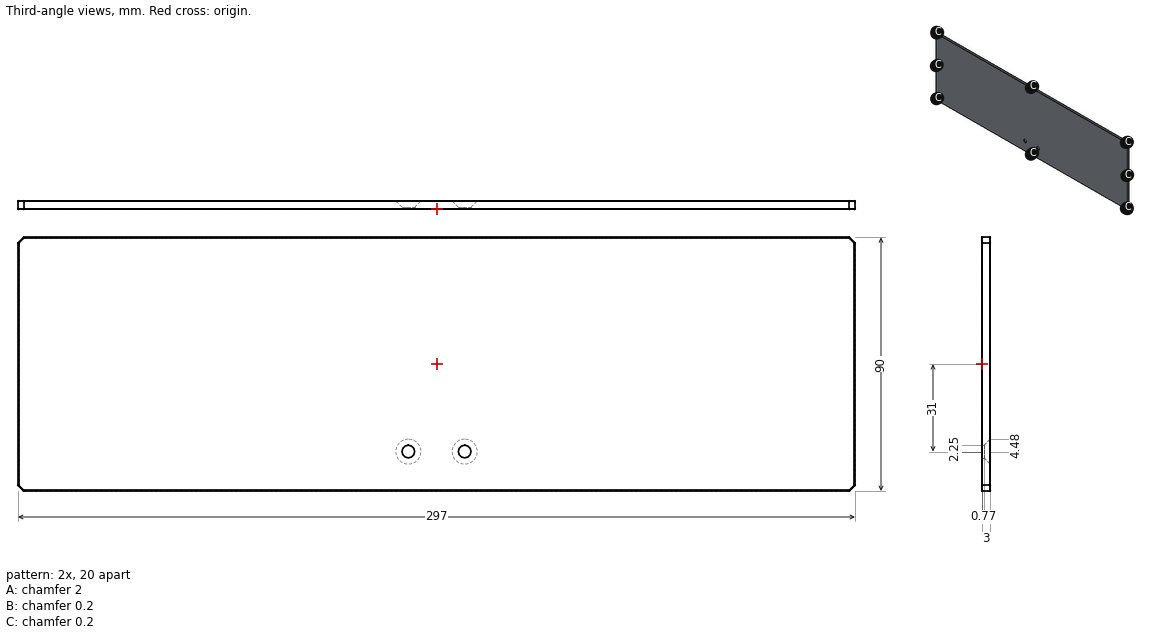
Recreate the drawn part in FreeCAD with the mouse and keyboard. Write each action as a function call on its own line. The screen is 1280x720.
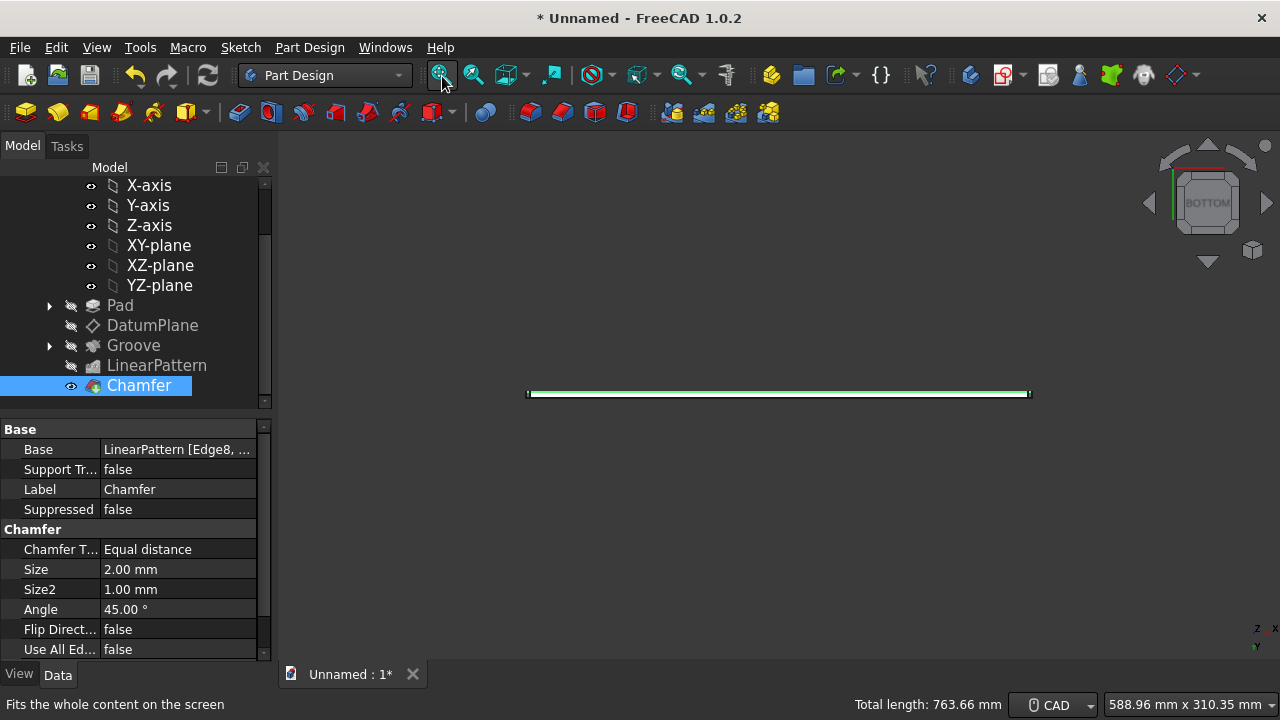
key(4)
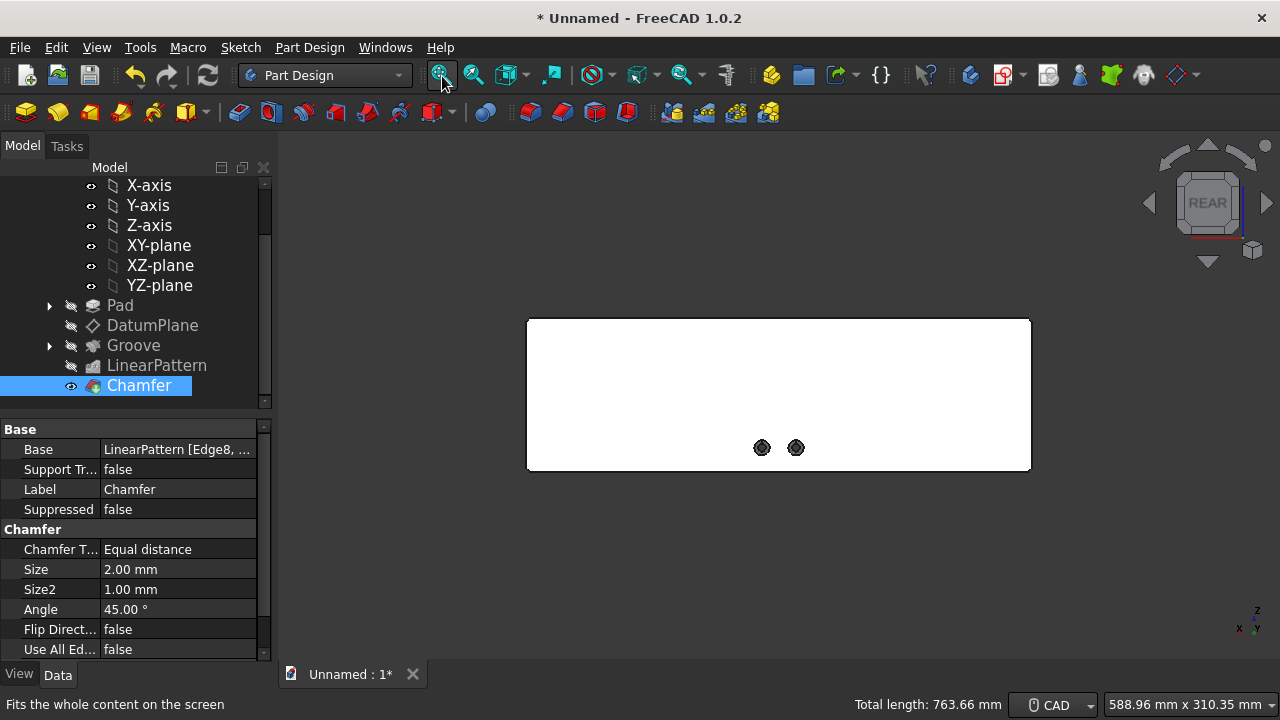
scroll(1030, 319, up, 11)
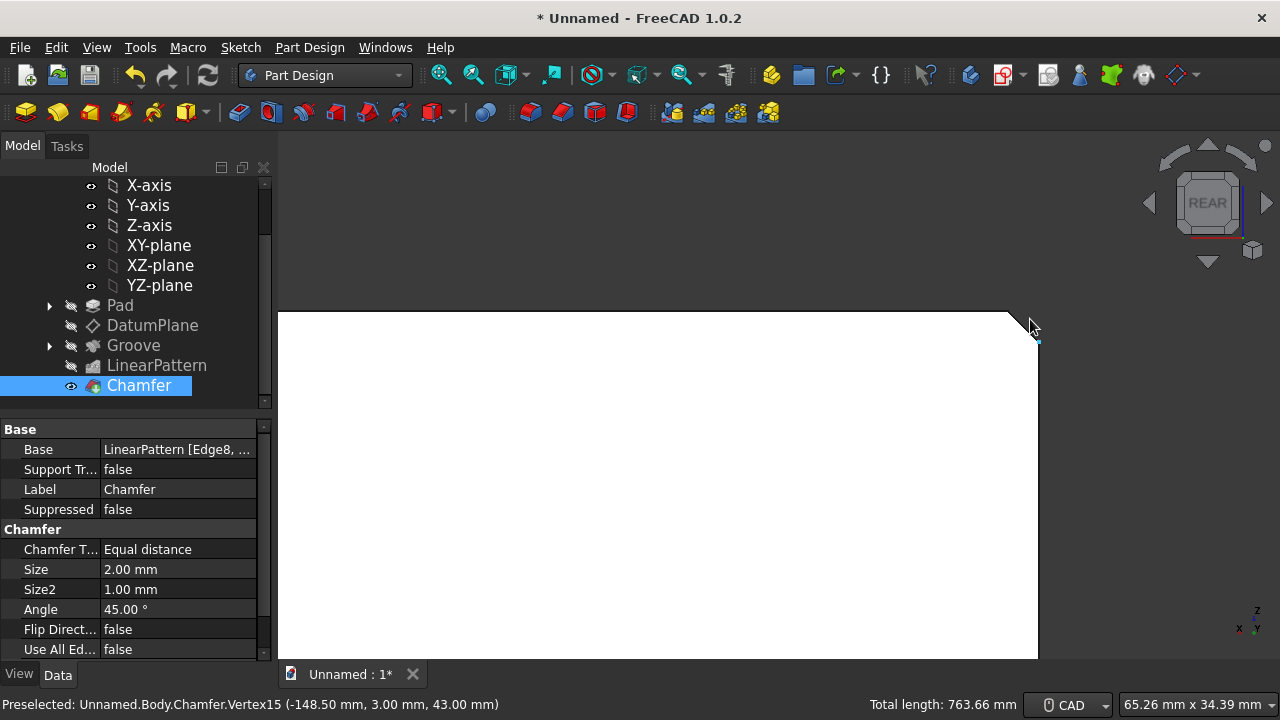
key(v)
key(f)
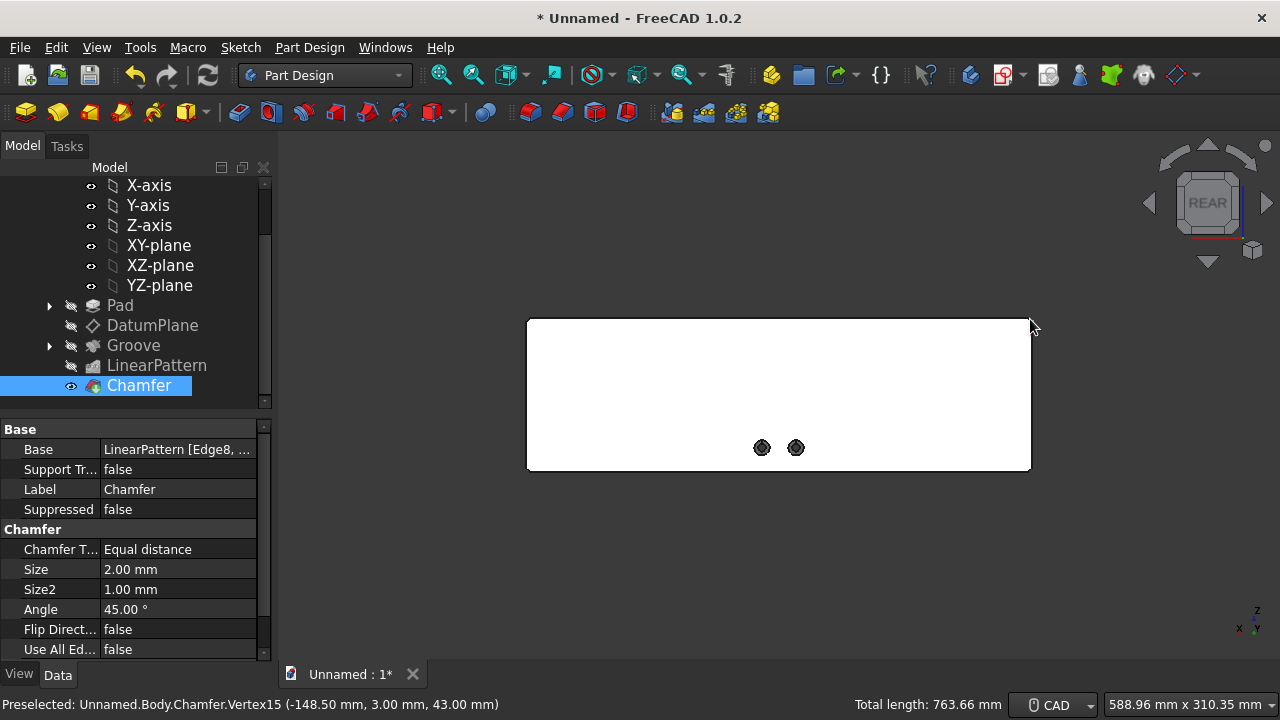
key(6)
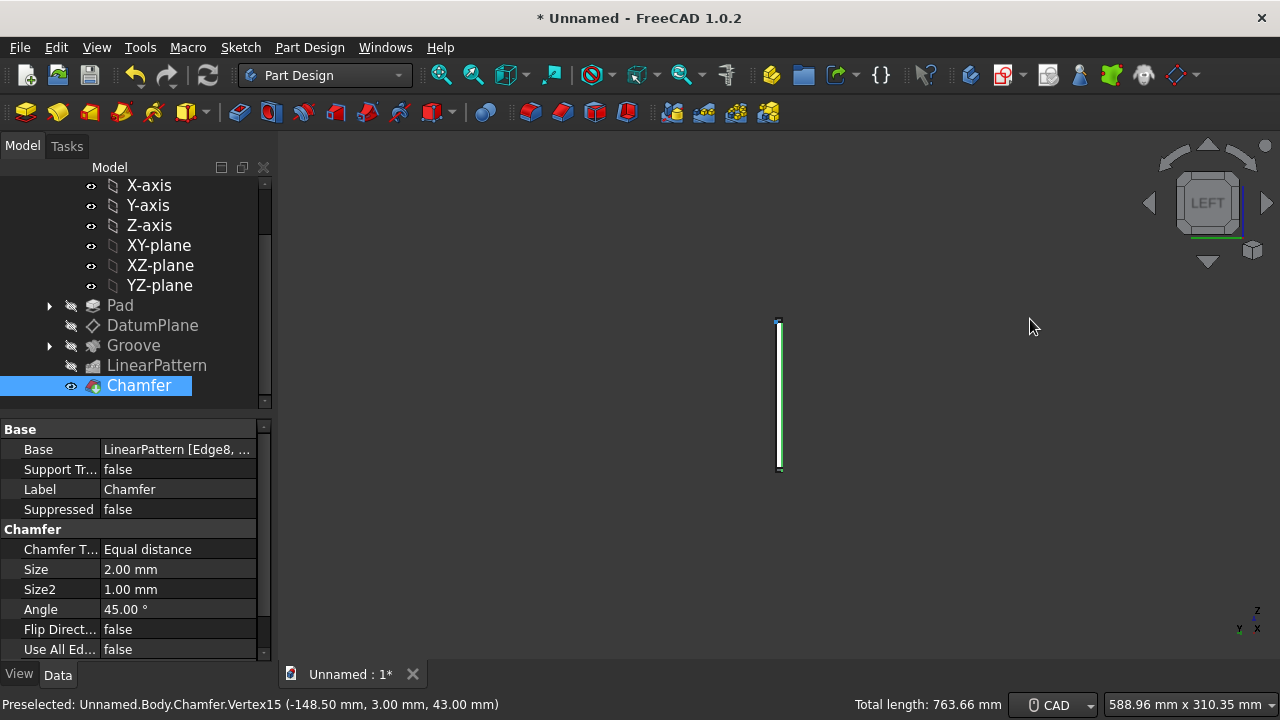
click(442, 76)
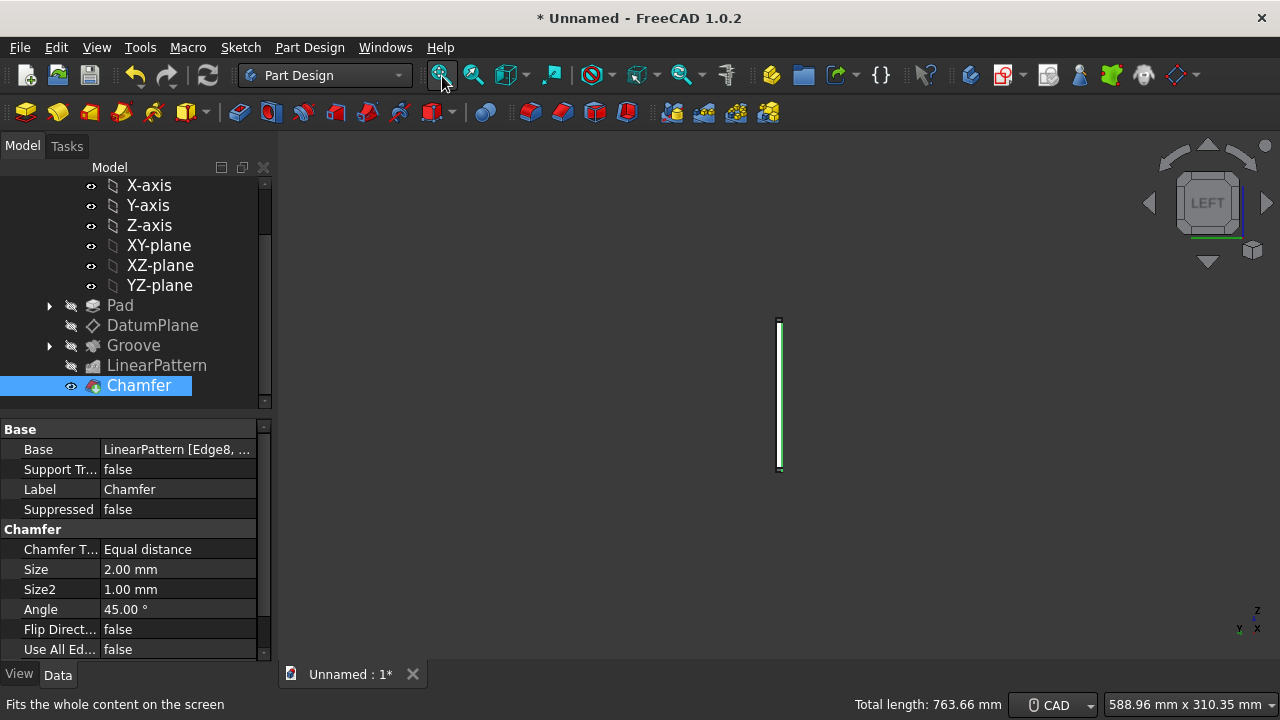
scroll(782, 319, up, 11)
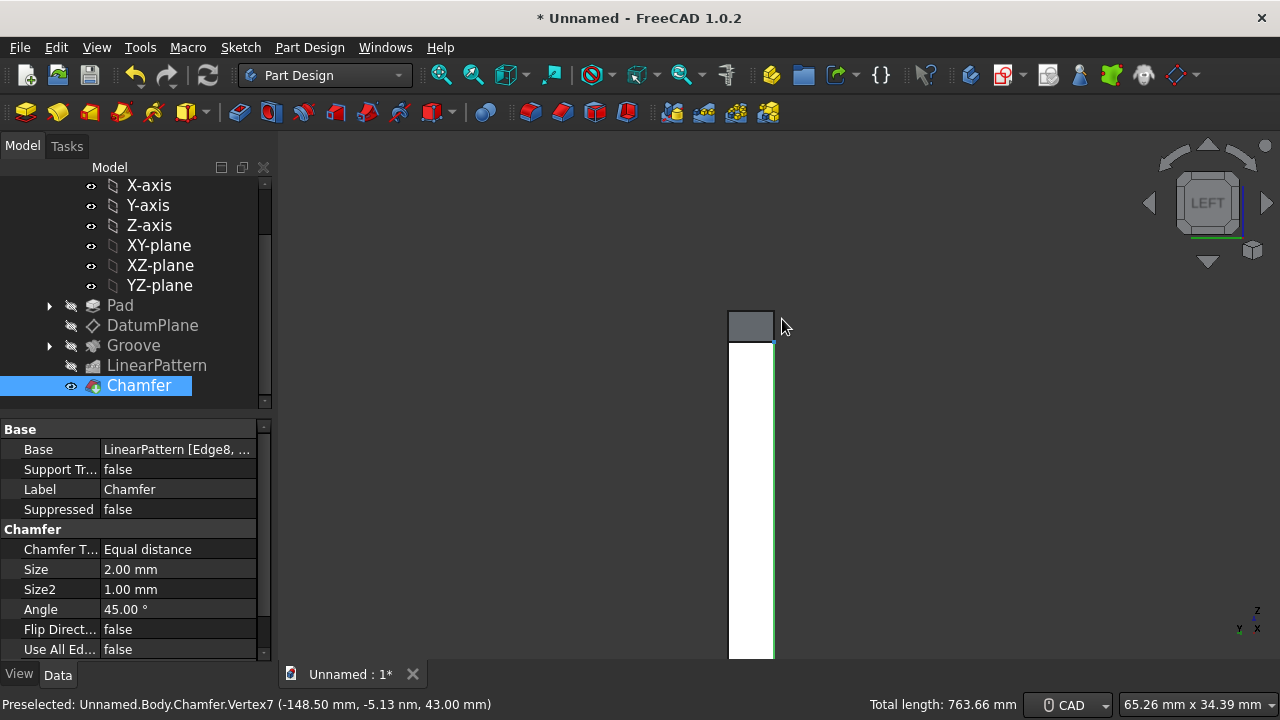
click(774, 325, ctrl)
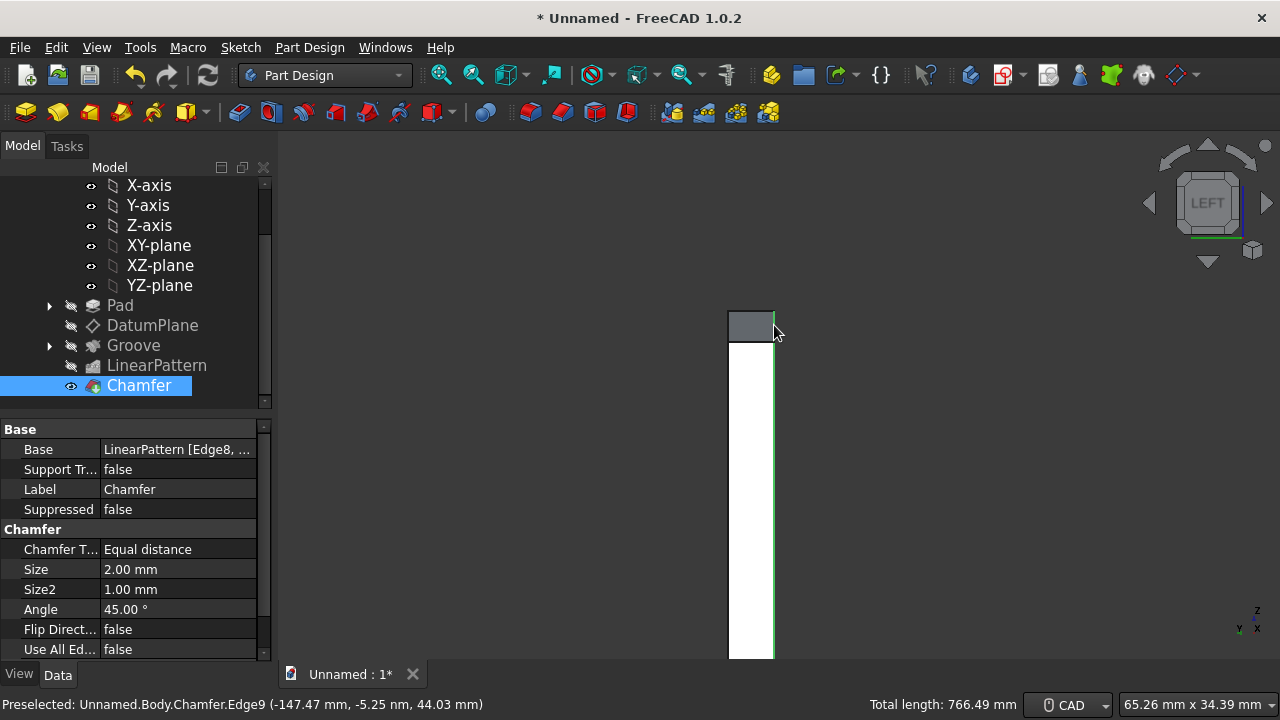
key(v)
key(f)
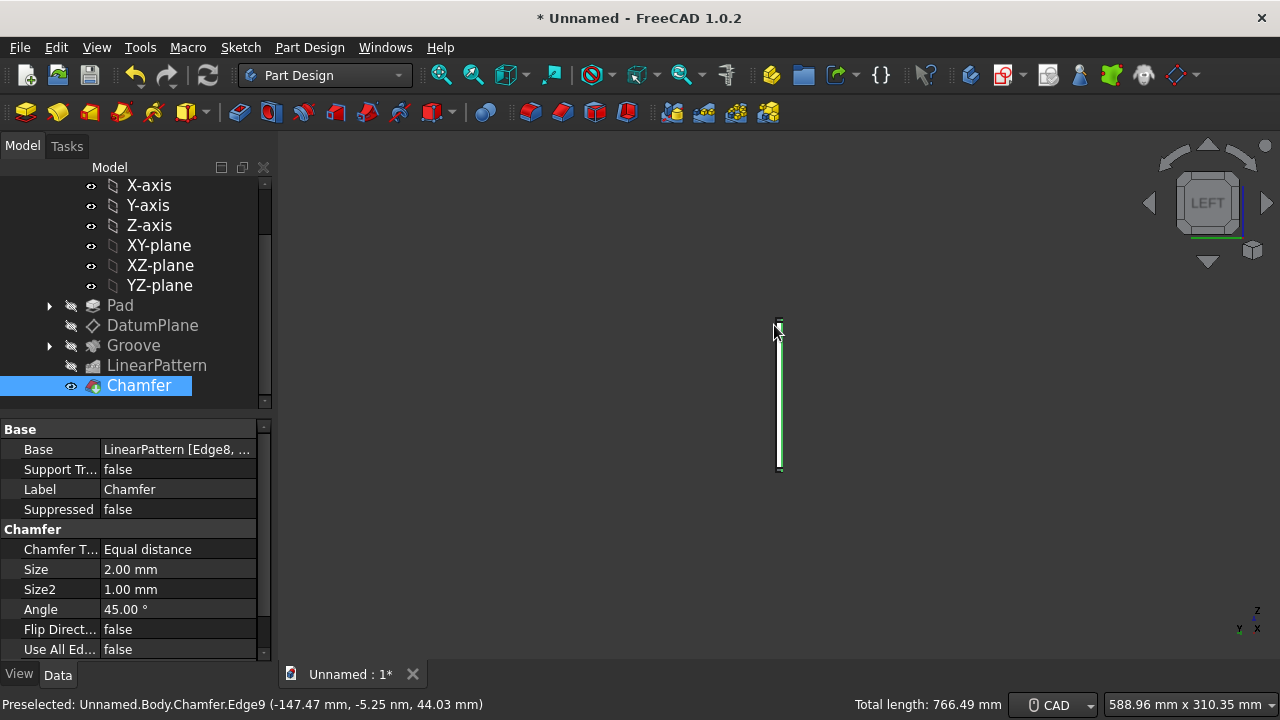
key(v)
key(3)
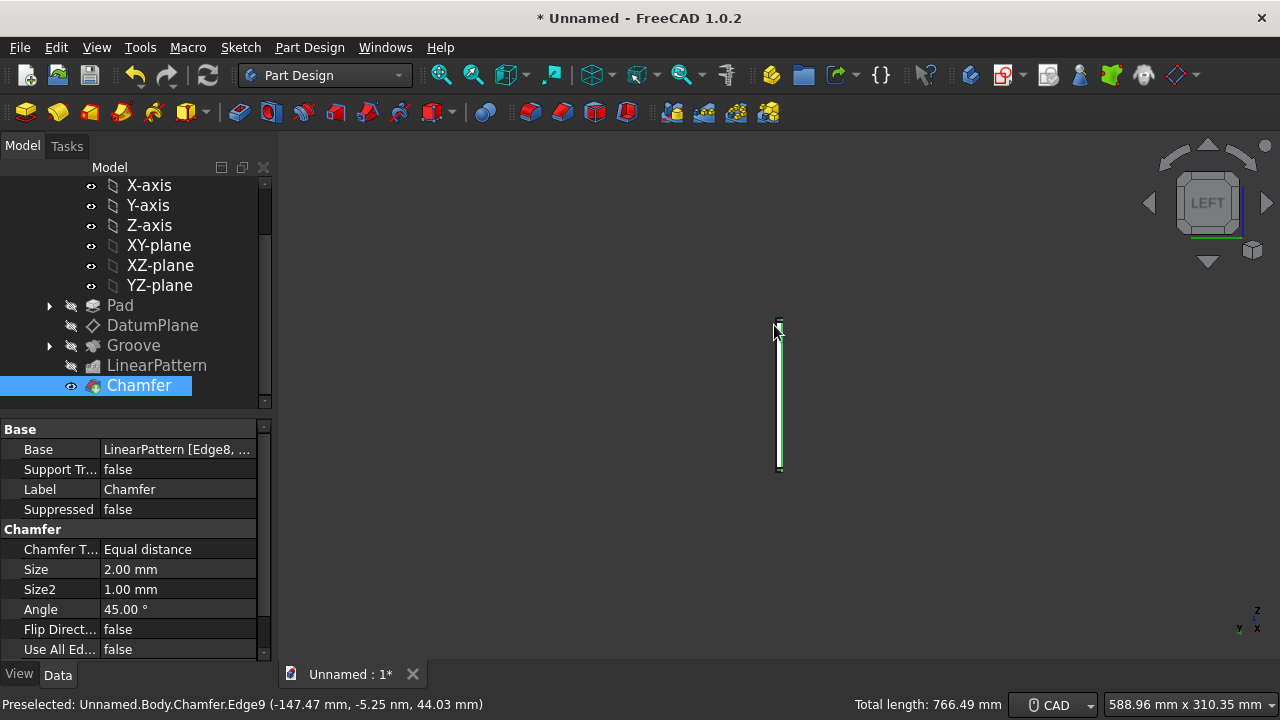
key(0)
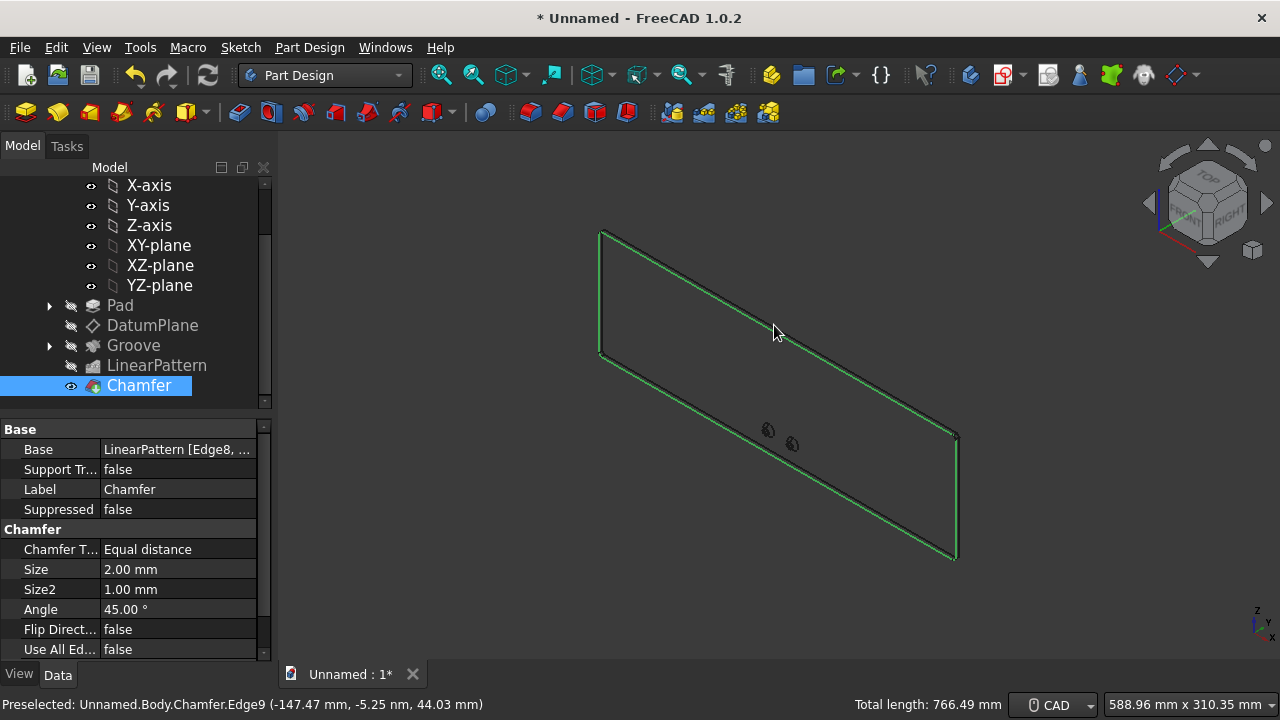
scroll(955, 436, up, 11)